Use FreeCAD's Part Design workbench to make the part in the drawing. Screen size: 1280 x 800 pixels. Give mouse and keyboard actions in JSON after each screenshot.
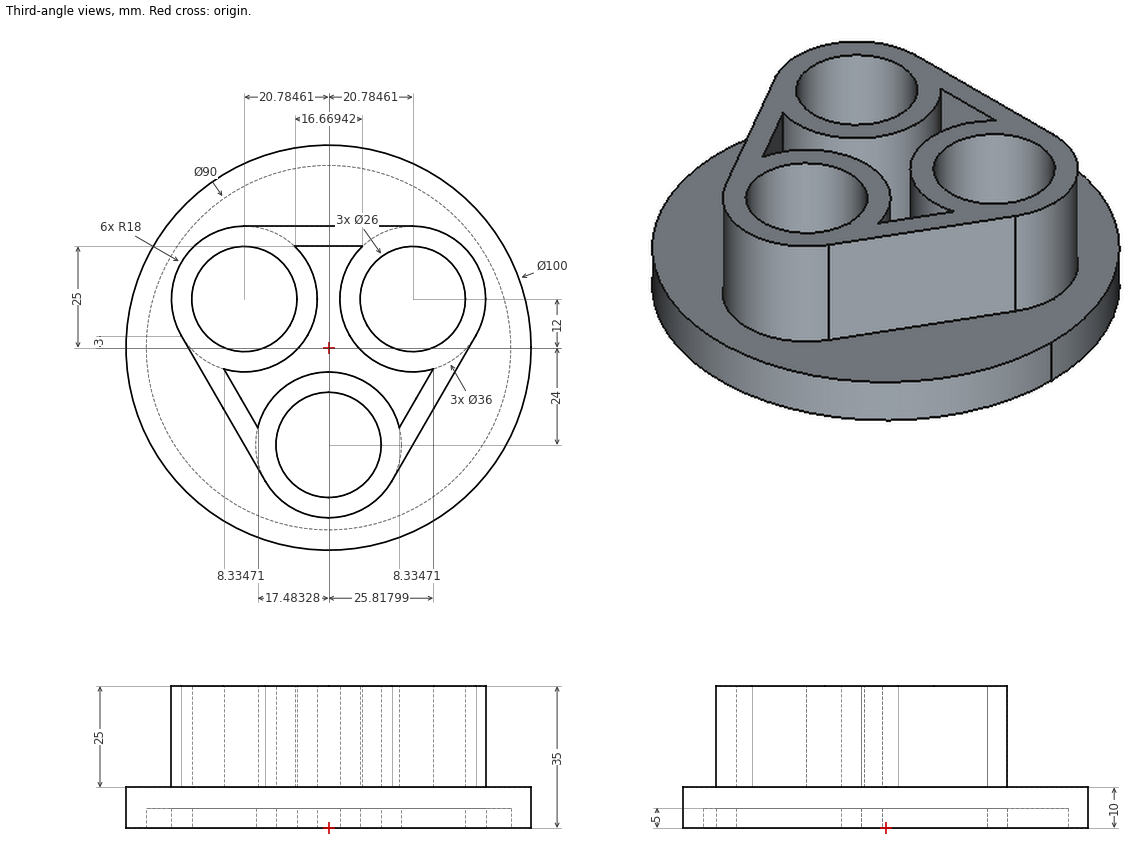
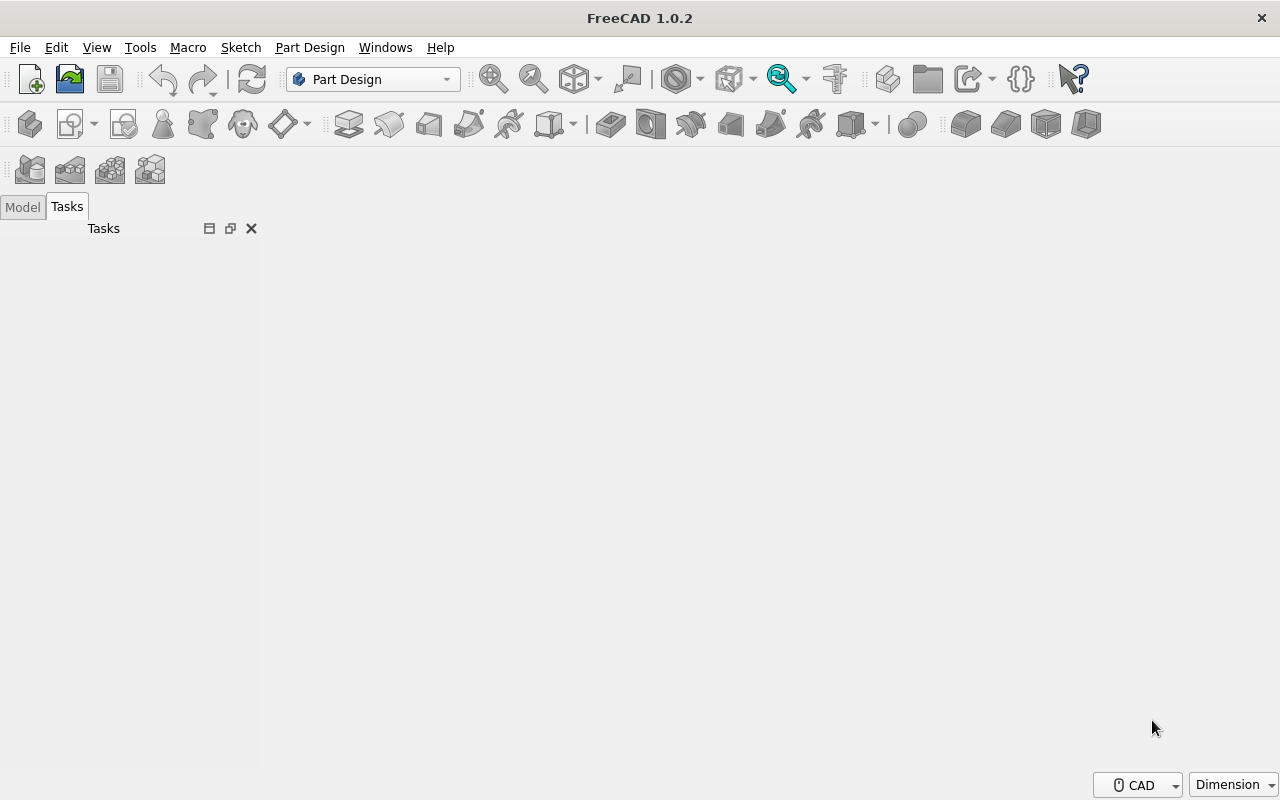
{"action": "left_click", "coordinate": [30, 80]}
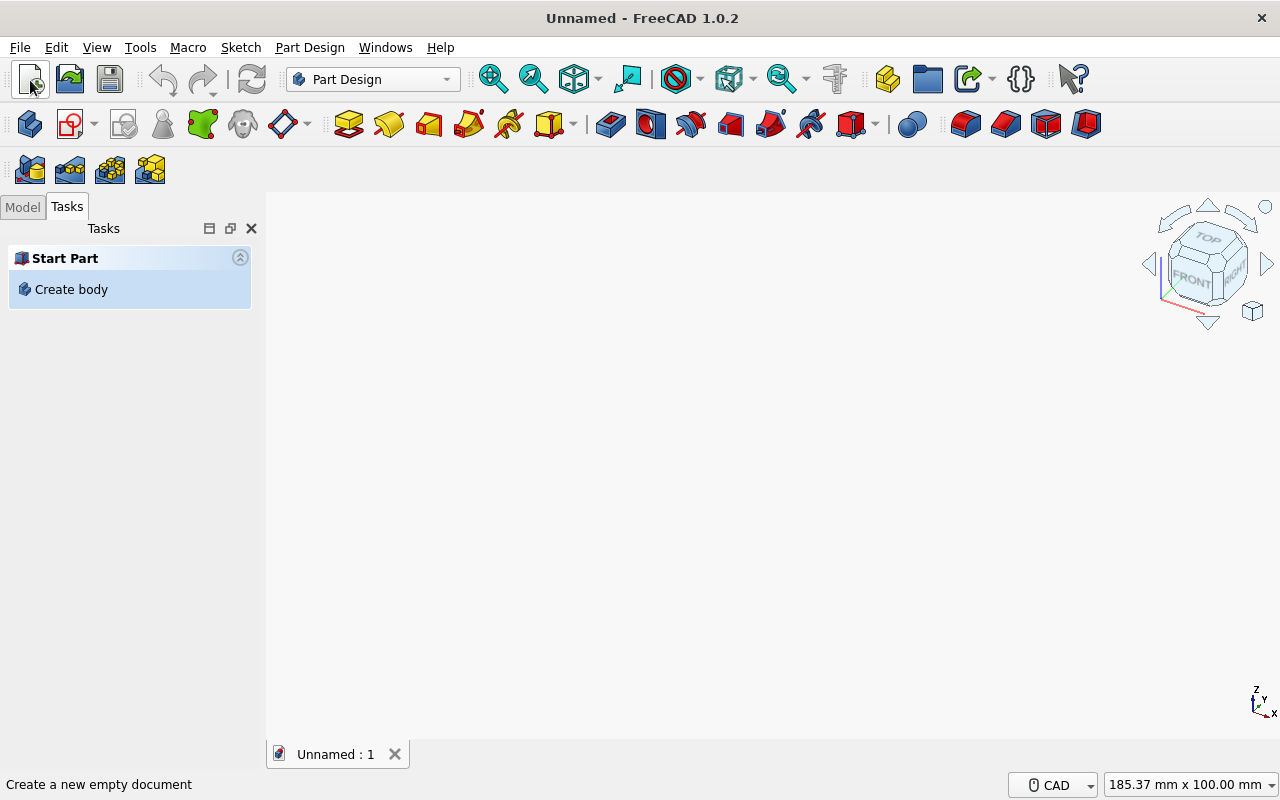
{"action": "left_click", "coordinate": [70, 124]}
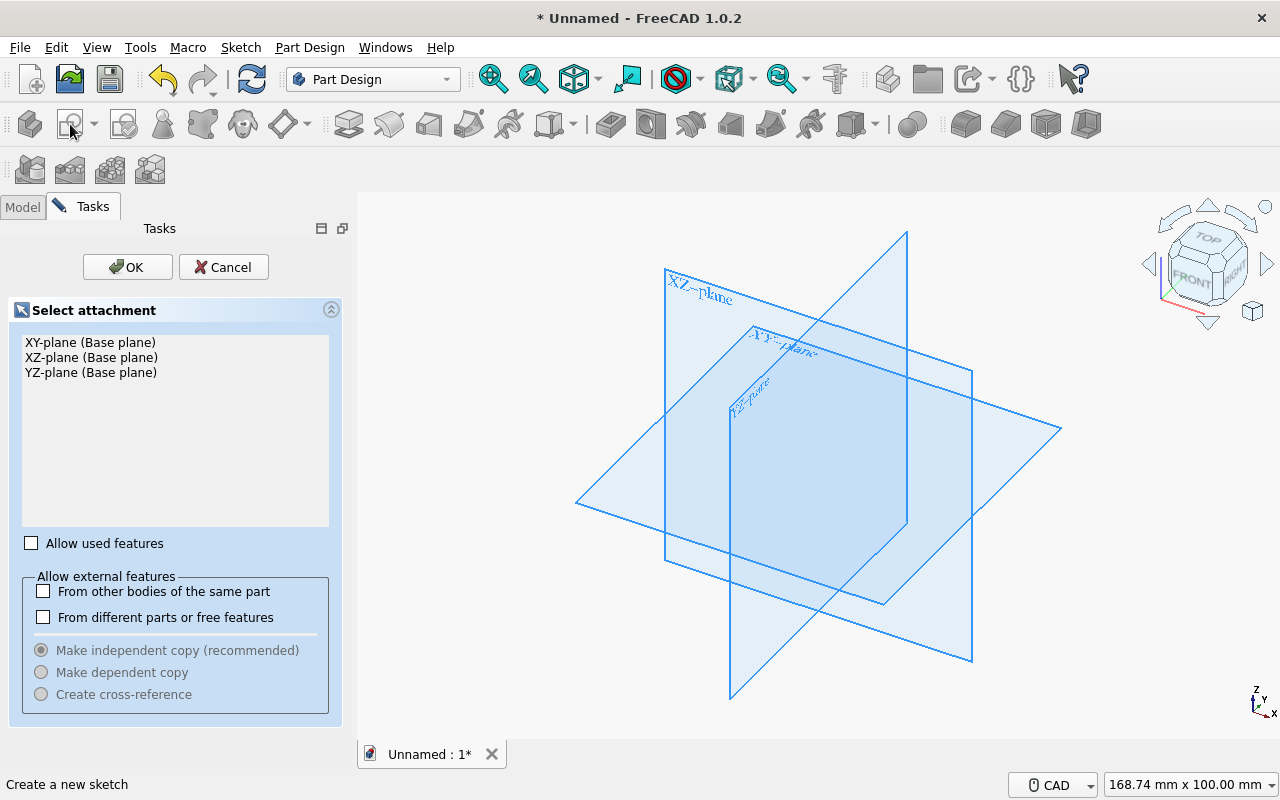
{"action": "left_click", "coordinate": [82, 342]}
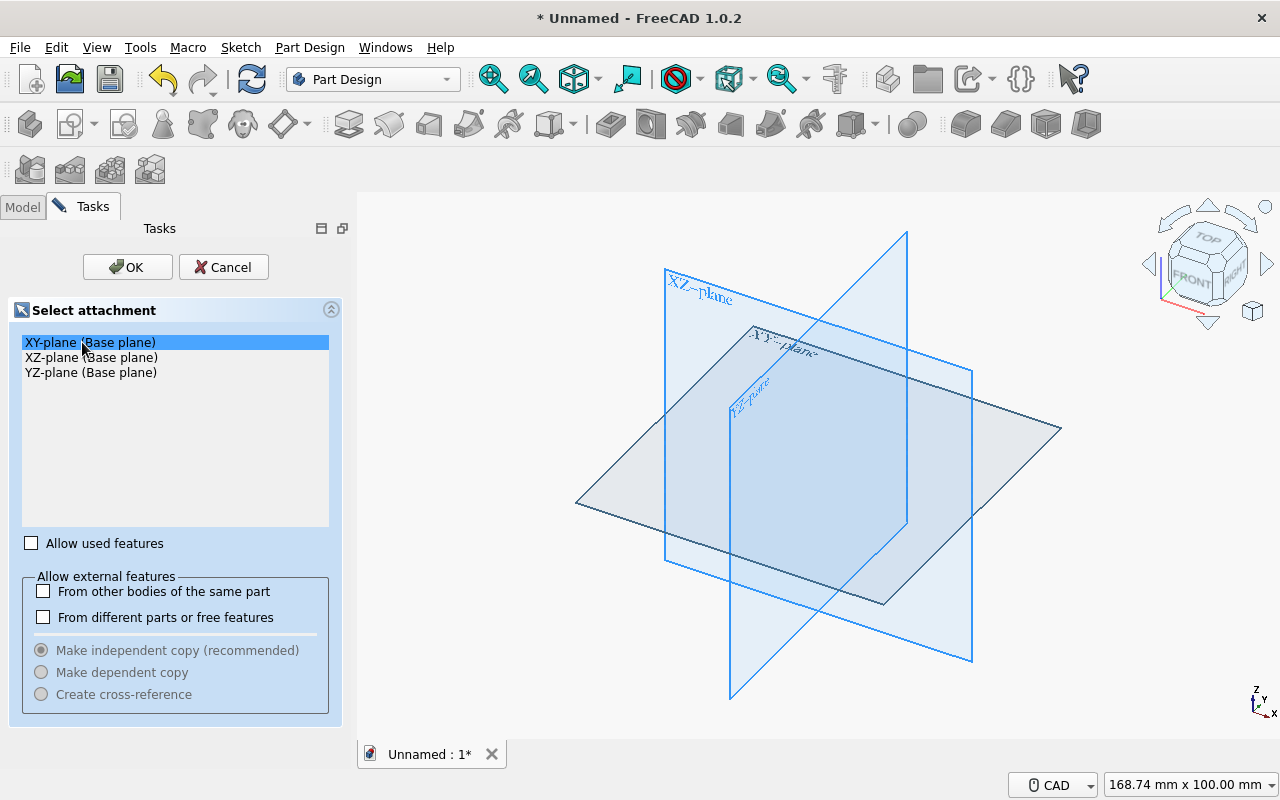
{"action": "left_click", "coordinate": [128, 267]}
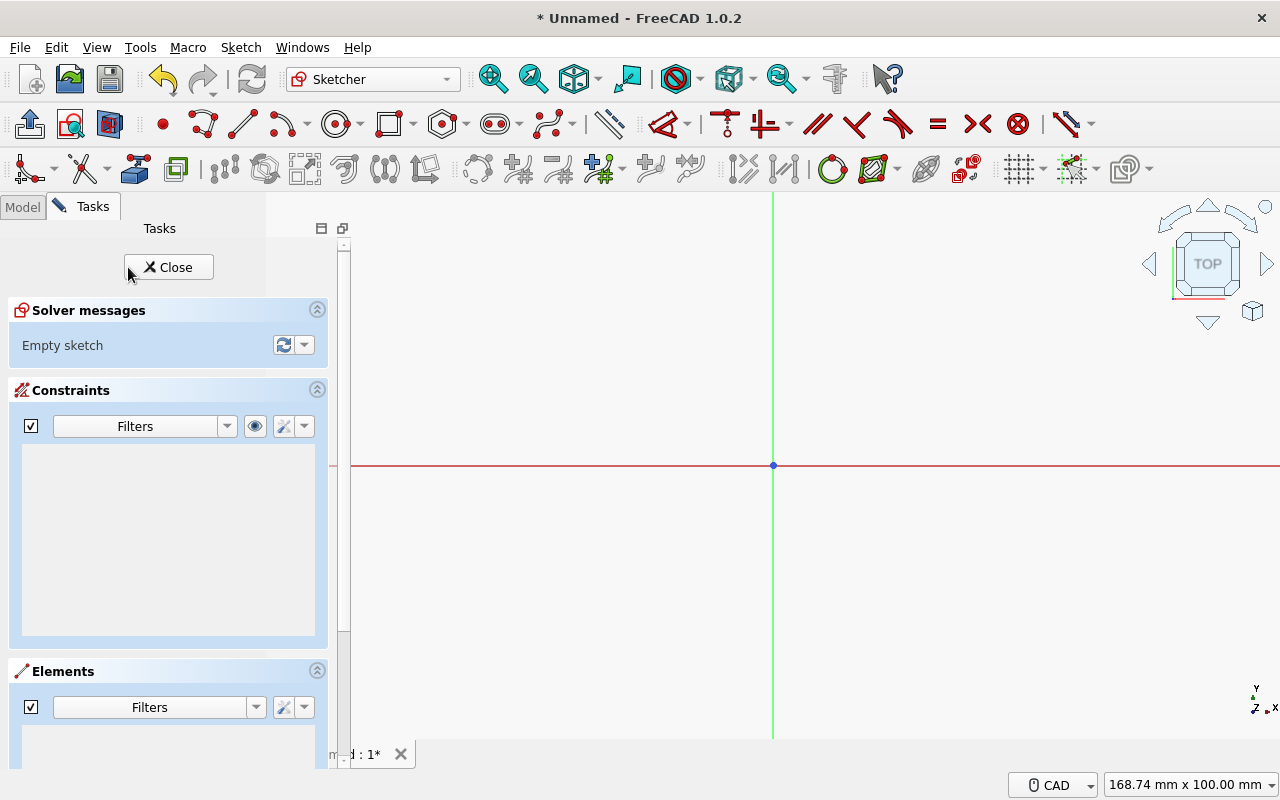
{"action": "scroll", "coordinate": [565, 466], "scroll_direction": "down", "scroll_amount": 2}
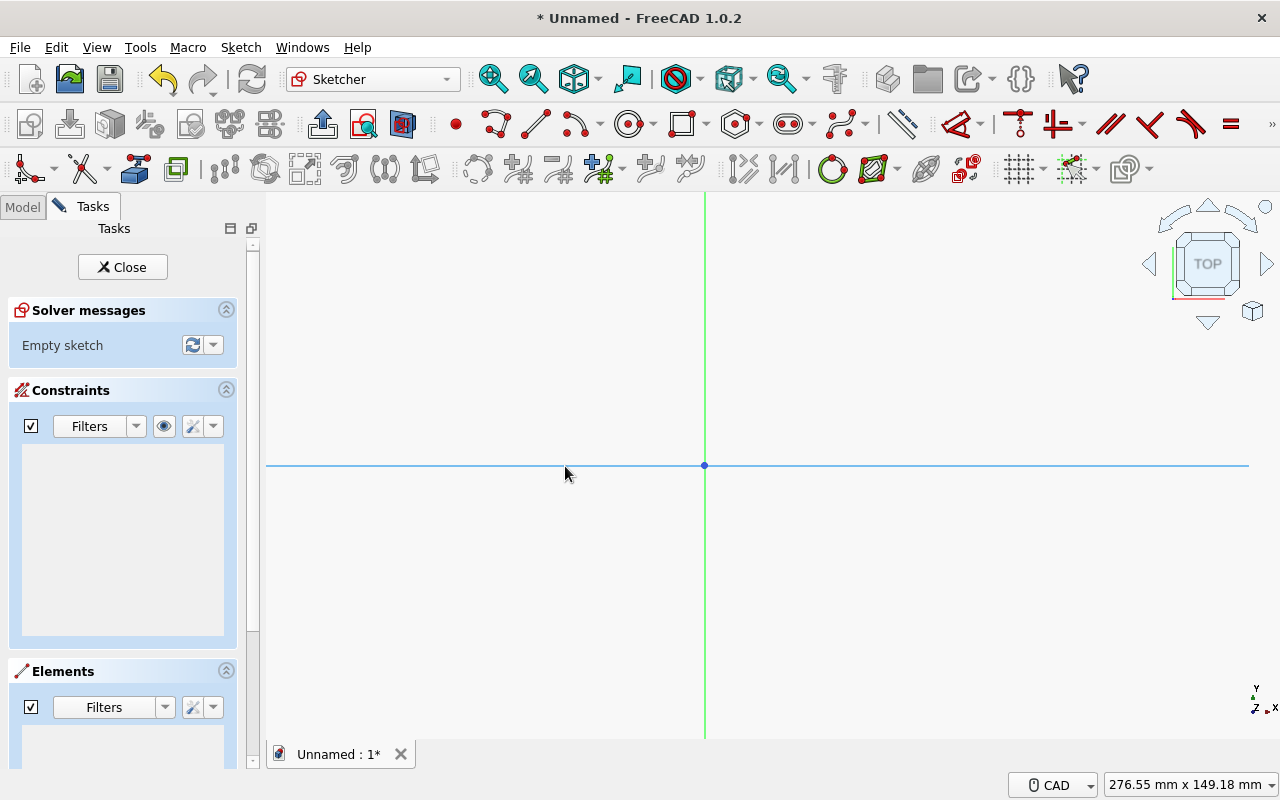
{"action": "left_click", "coordinate": [630, 124]}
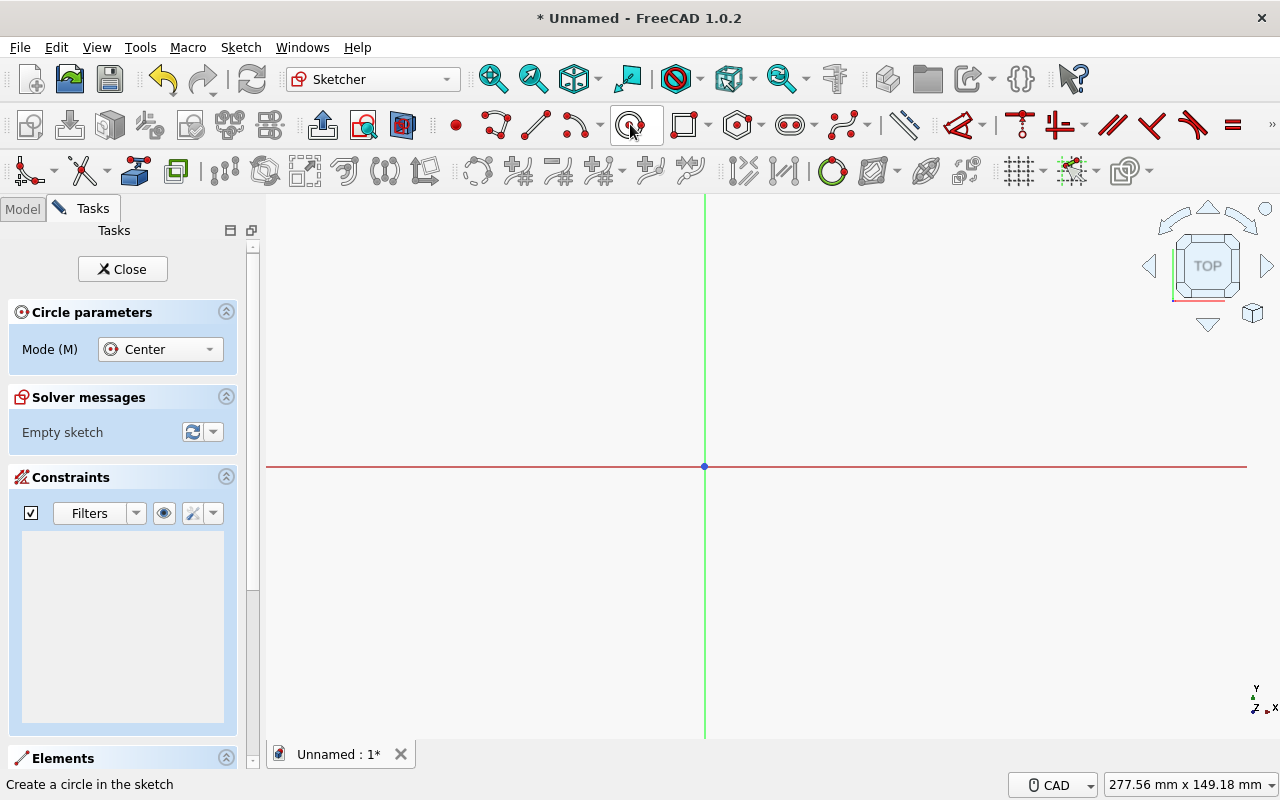
{"action": "left_click", "coordinate": [705, 467]}
{"action": "left_click", "coordinate": [834, 338]}
{"action": "key", "text": "Escape"}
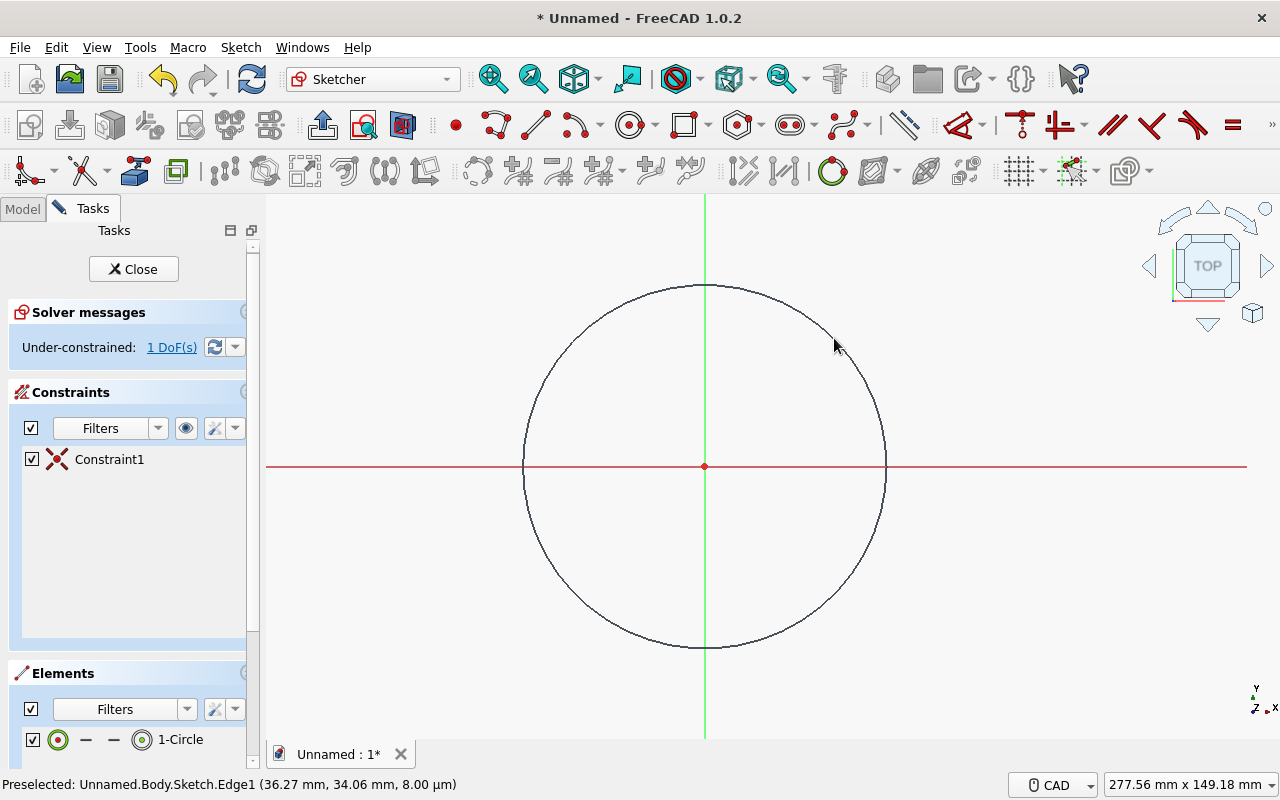
{"action": "left_click", "coordinate": [958, 126]}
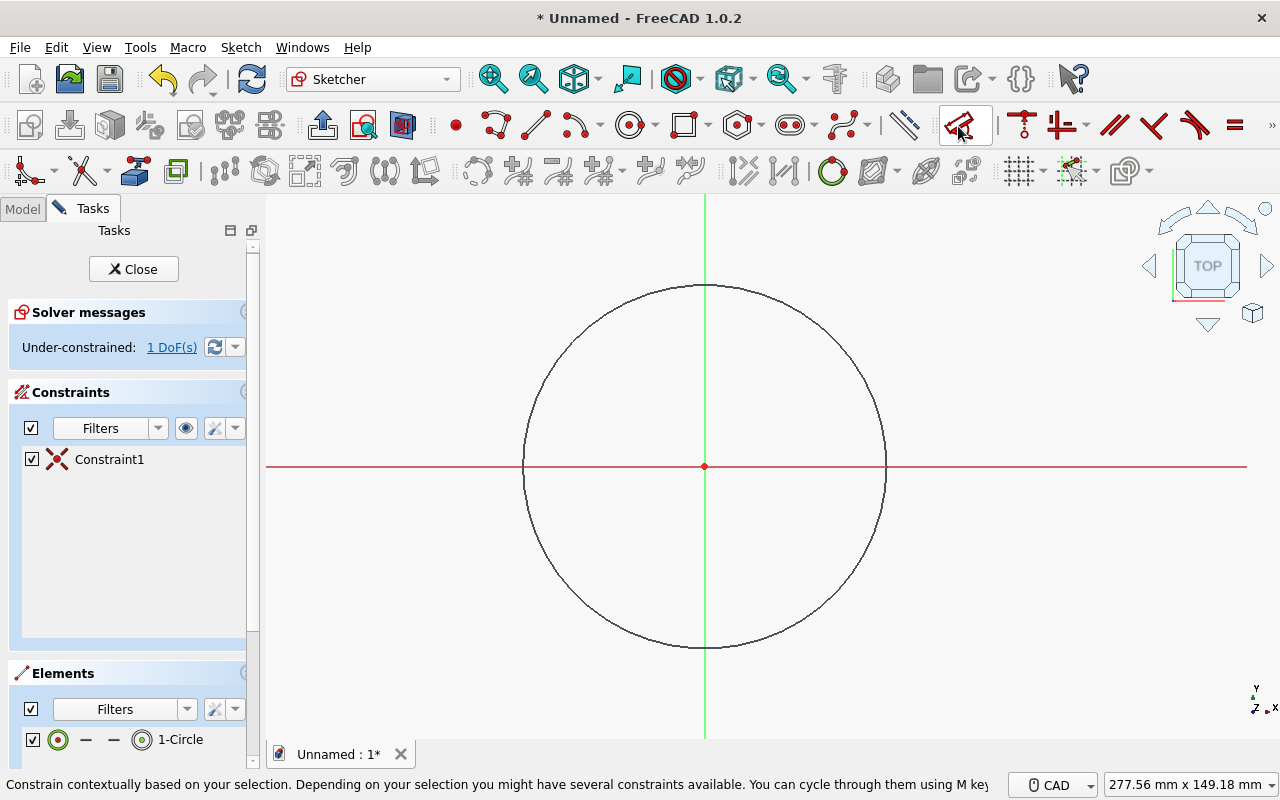
{"action": "left_click", "coordinate": [833, 338]}
{"action": "left_click", "coordinate": [856, 315]}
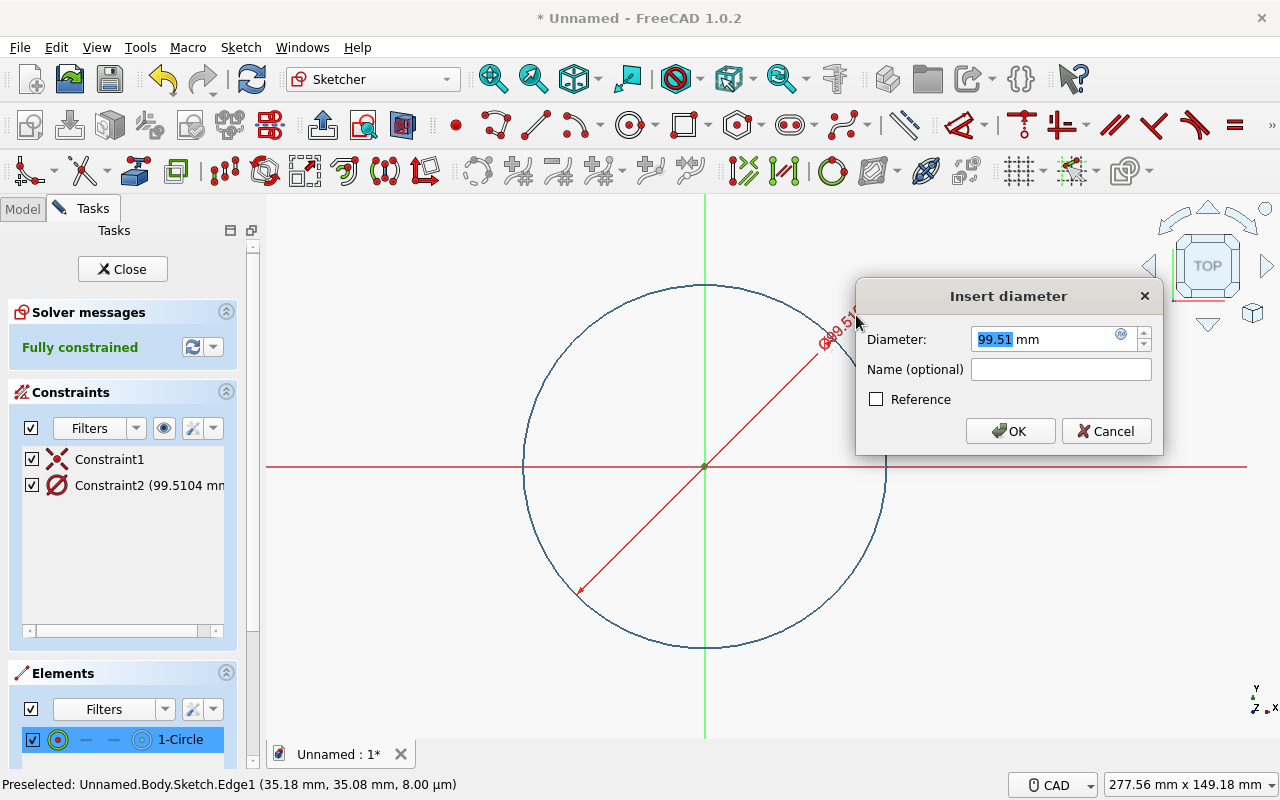
{"action": "type", "text": "100"}
{"action": "key", "text": "Return"}
{"action": "key", "text": "Escape"}